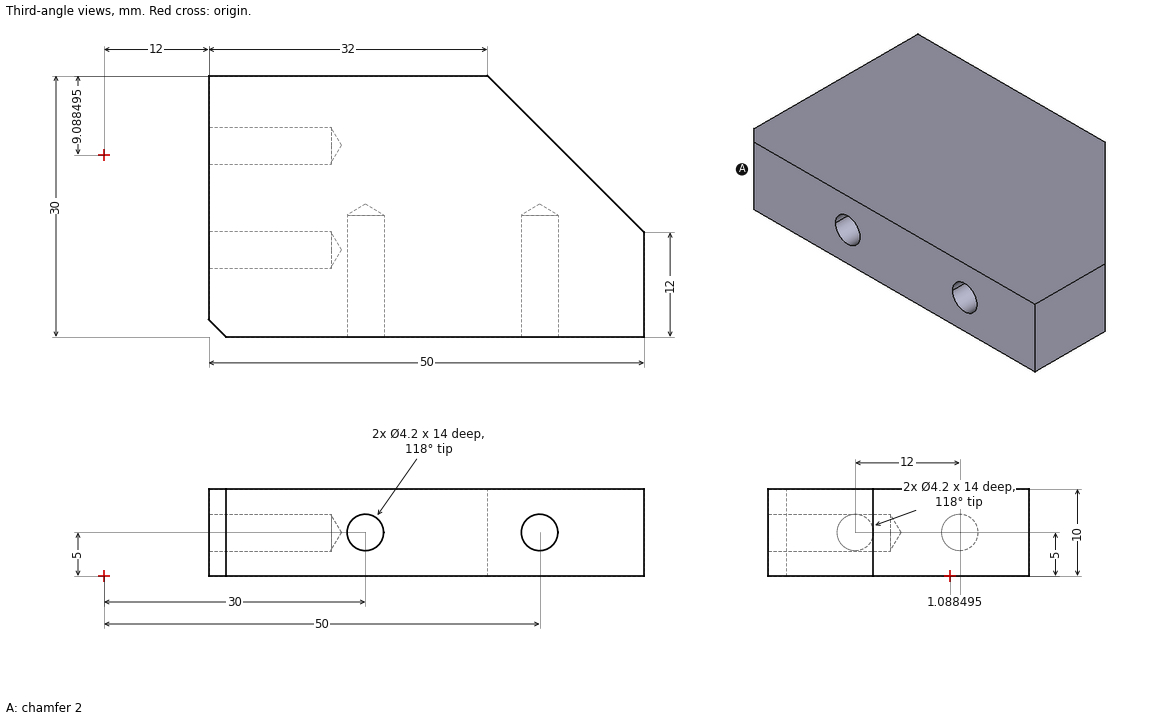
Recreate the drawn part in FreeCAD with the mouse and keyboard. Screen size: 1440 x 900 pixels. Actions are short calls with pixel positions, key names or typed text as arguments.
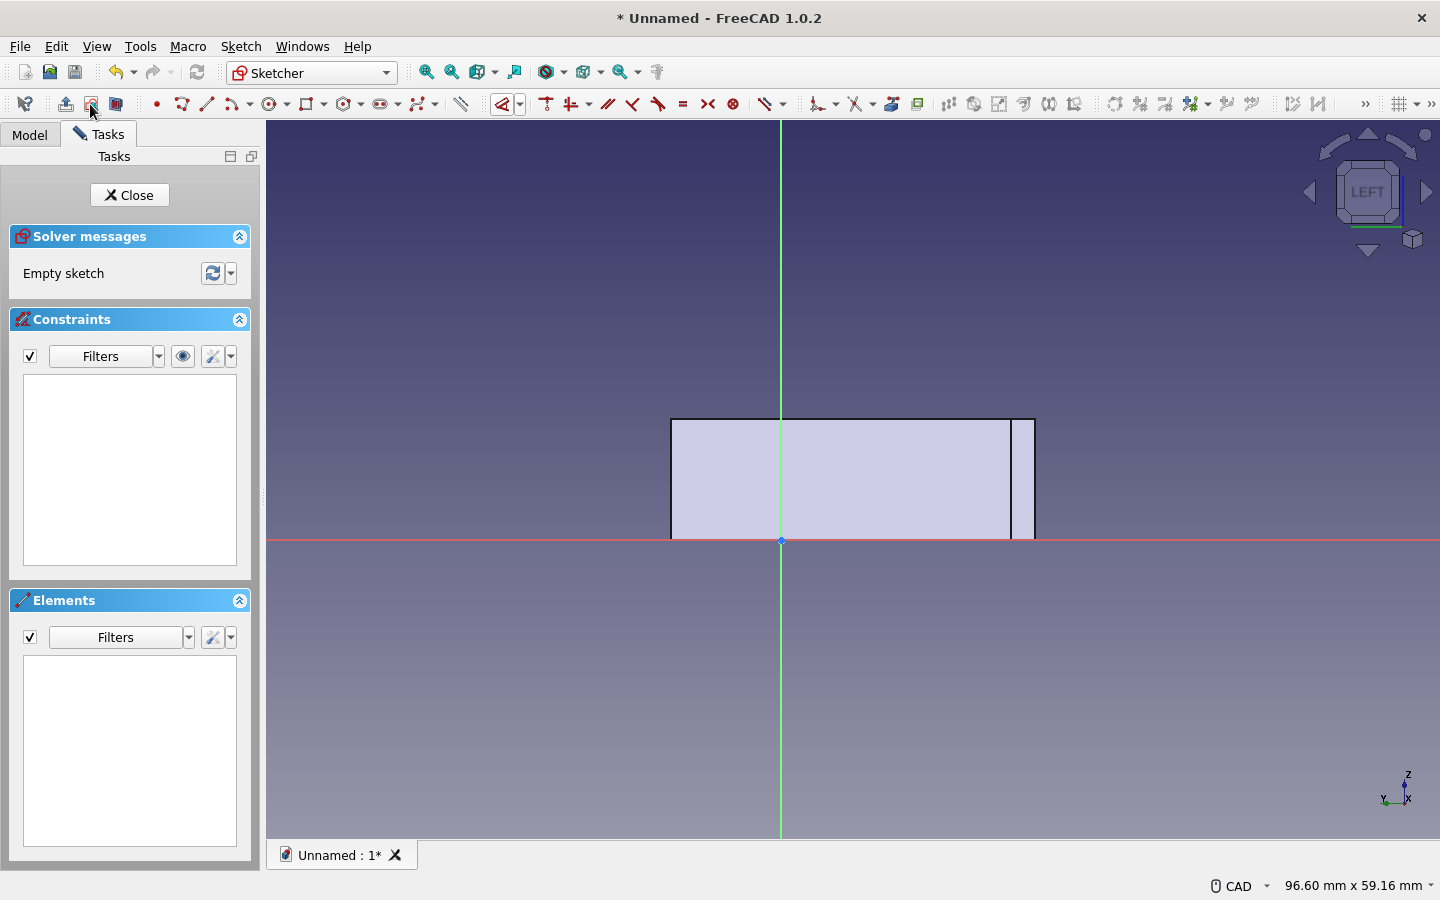
scroll(865, 505, up, 6)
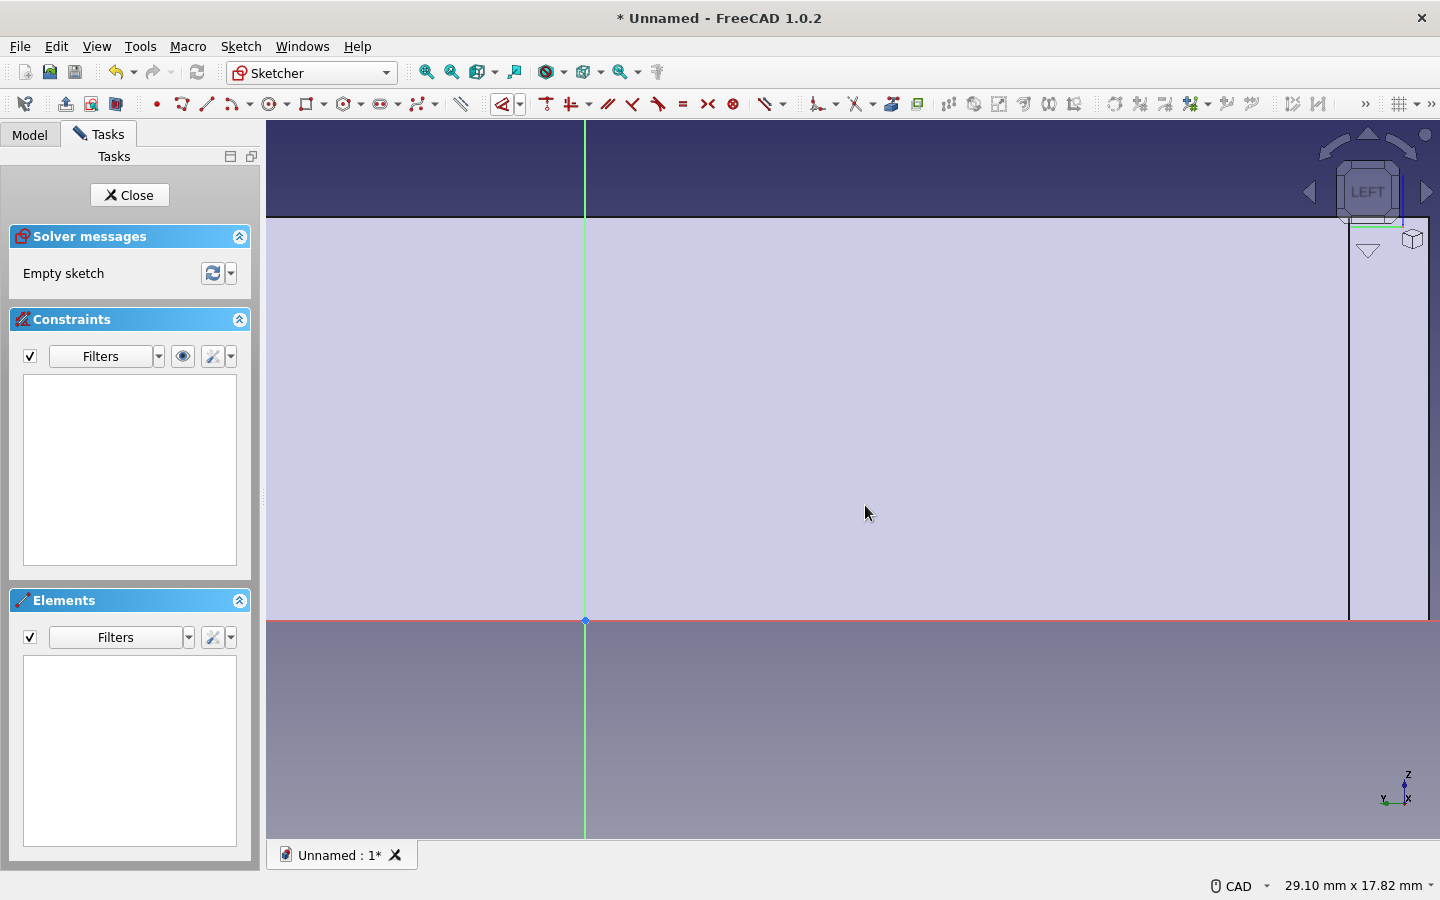
click(268, 104)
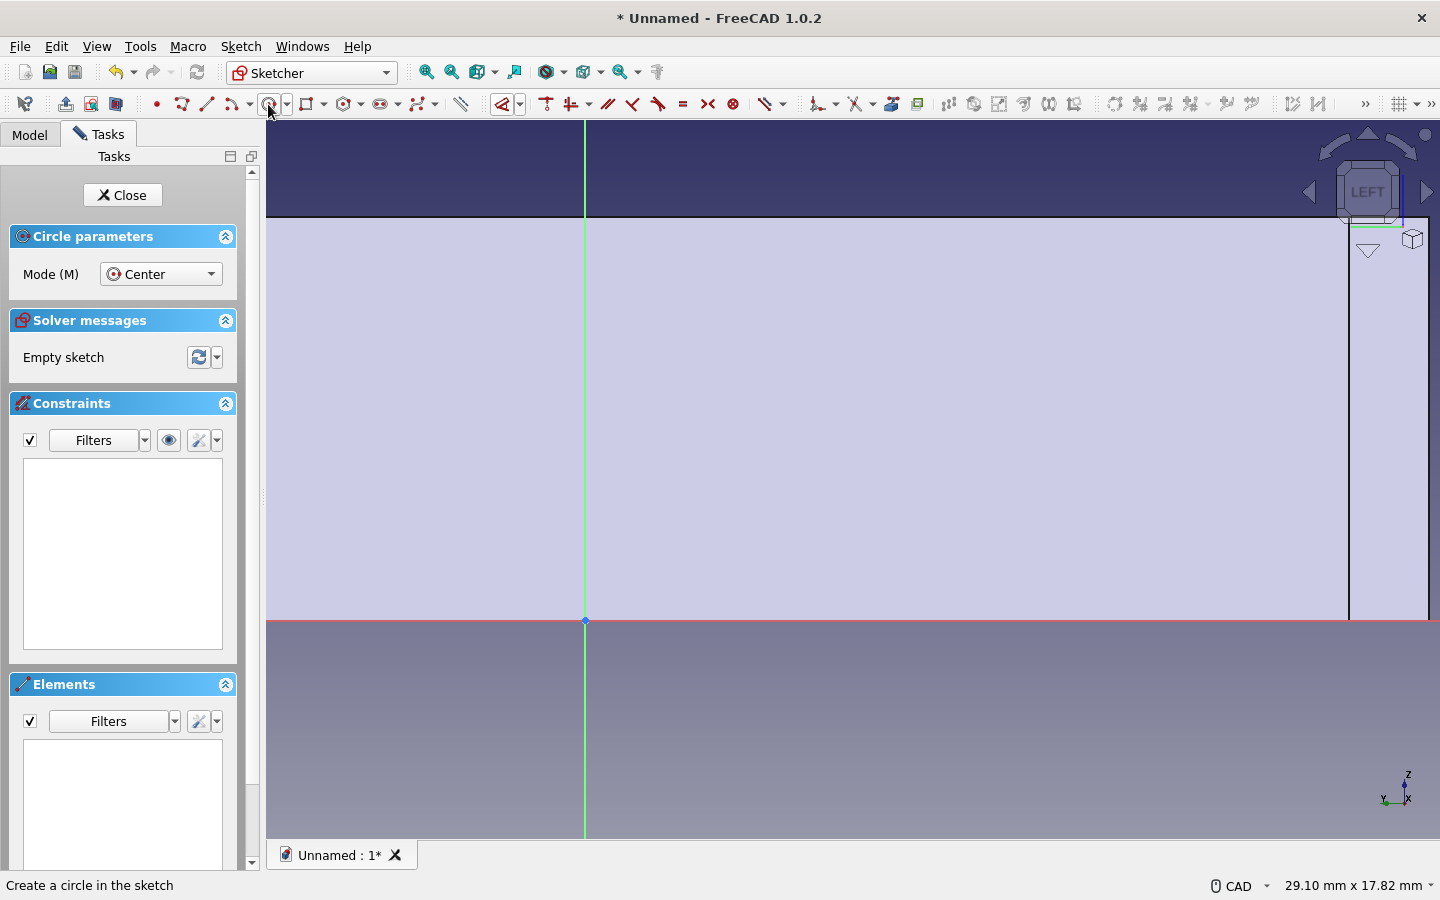
click(1026, 419)
move(1086, 359)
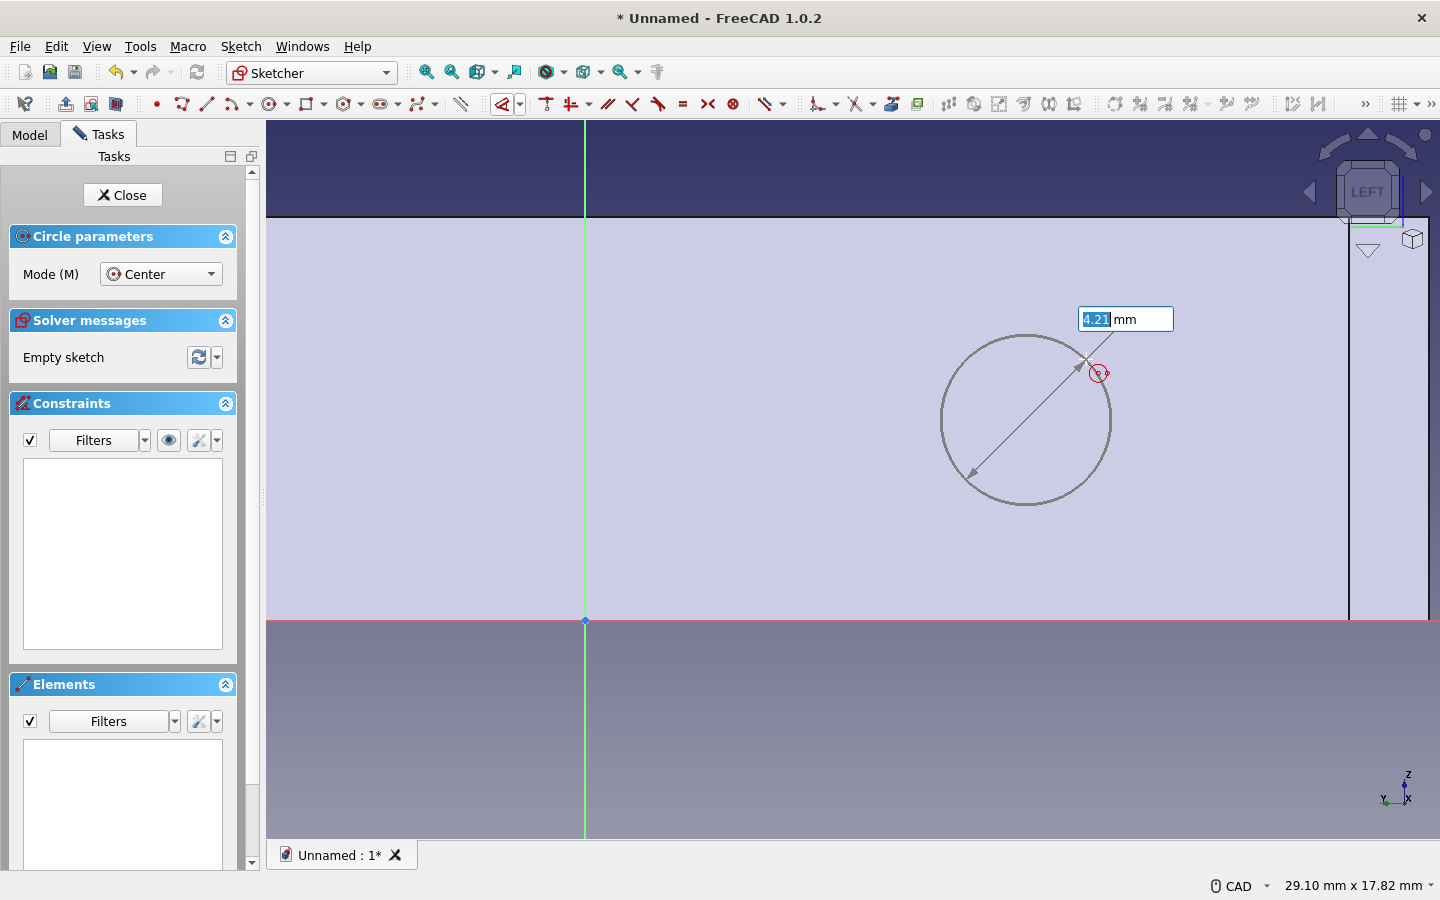
text(4.2)
key(Return)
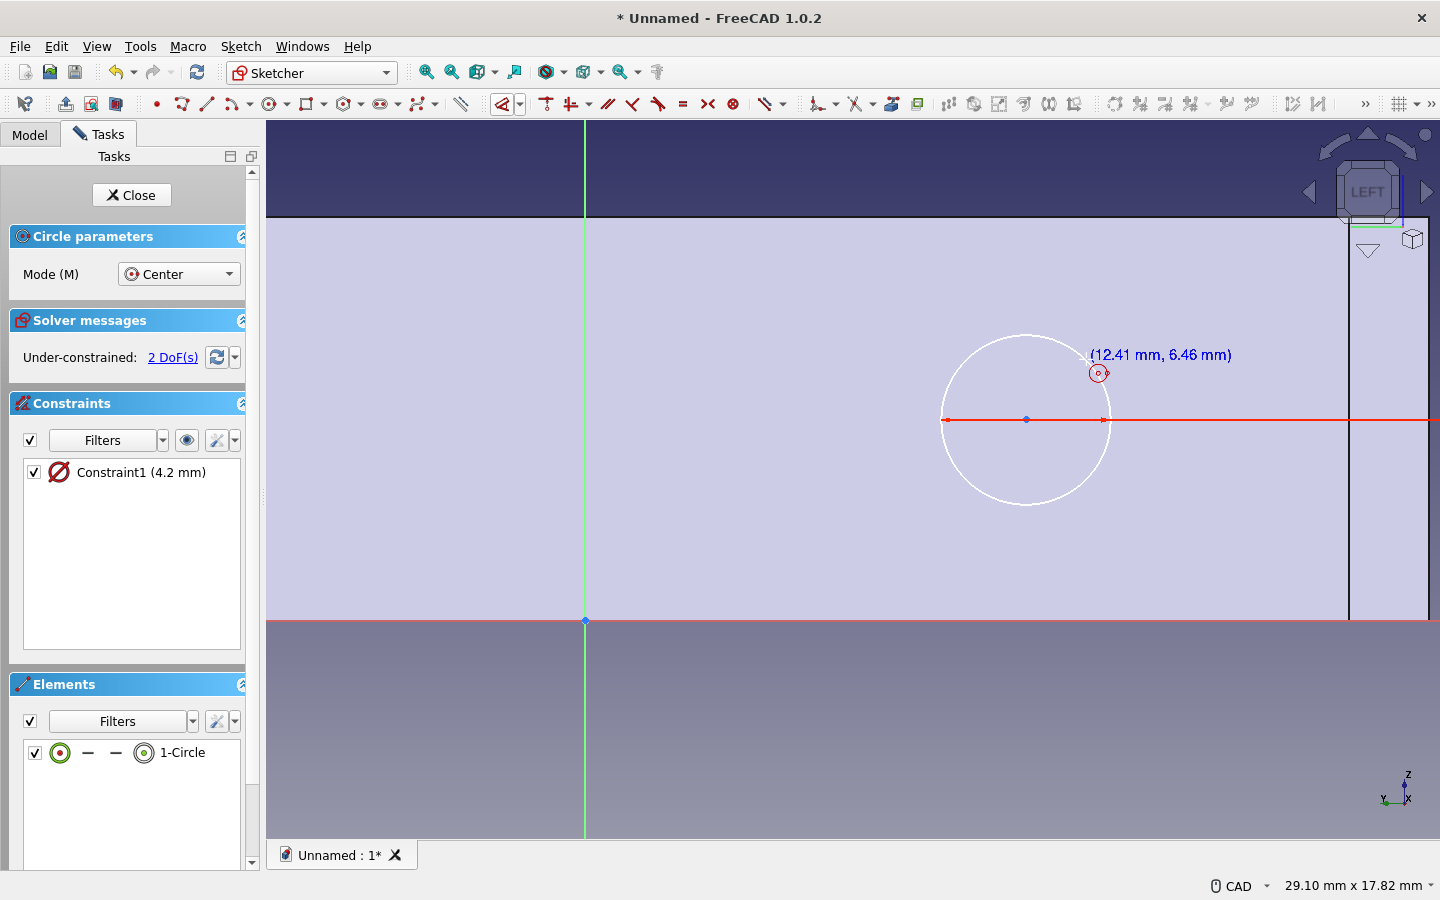
click(542, 419)
move(601, 359)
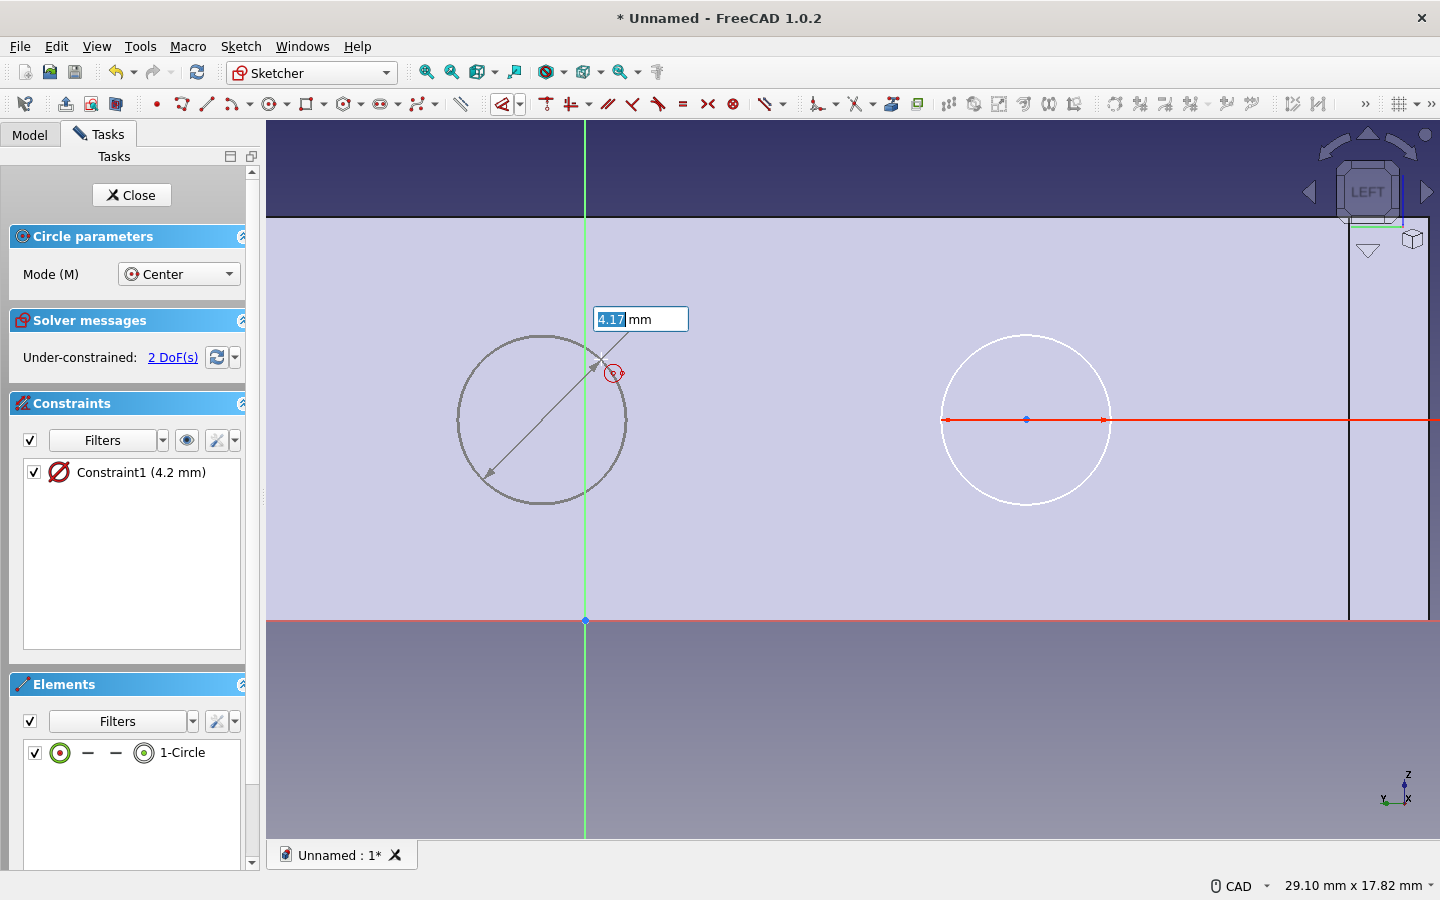
text(4.2)
key(Return)
key(Escape)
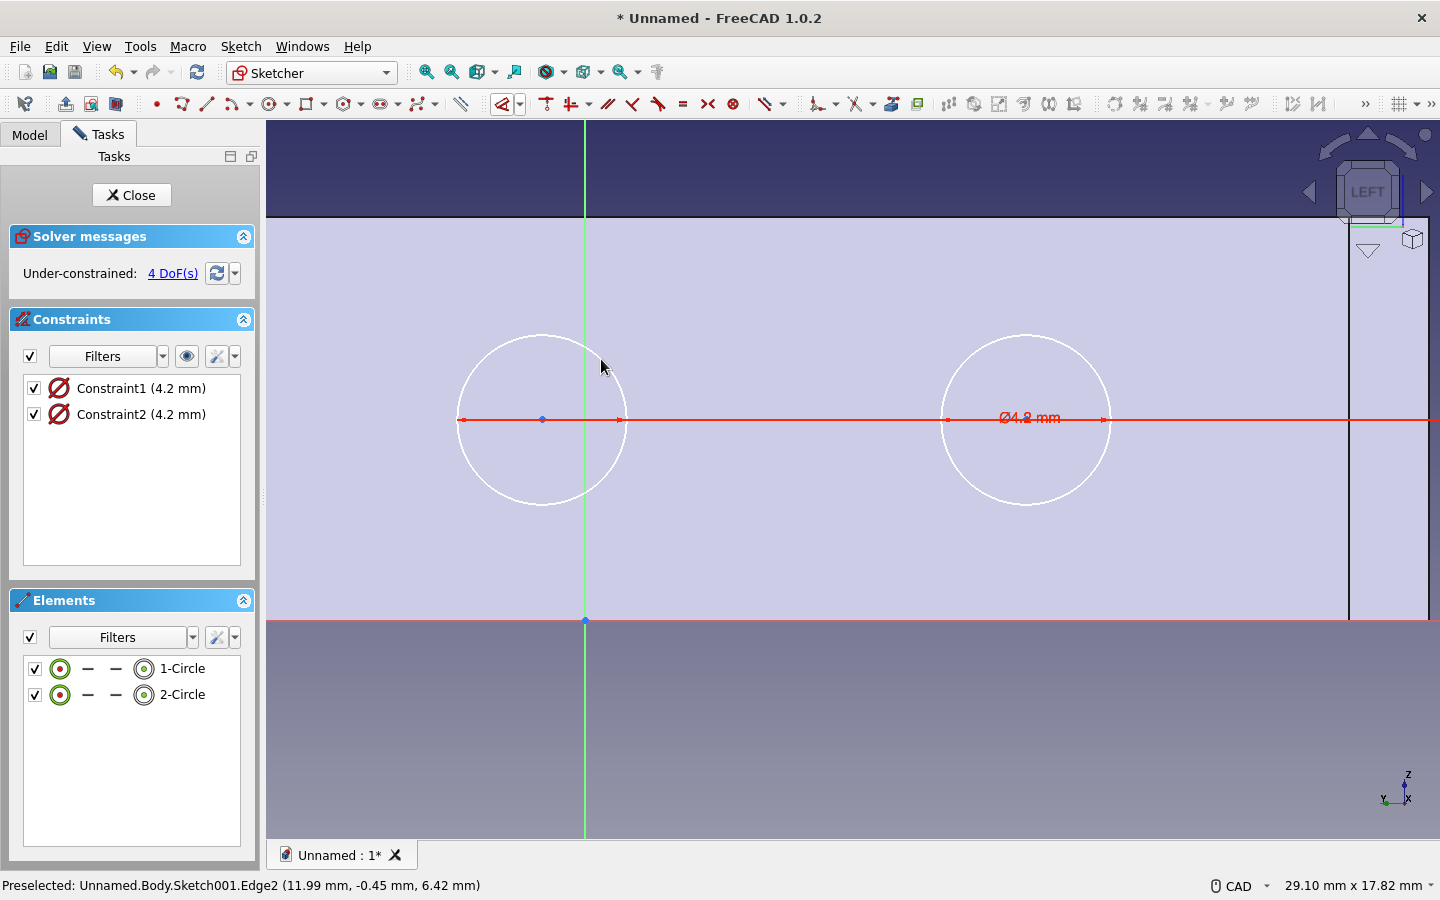
click(1026, 420)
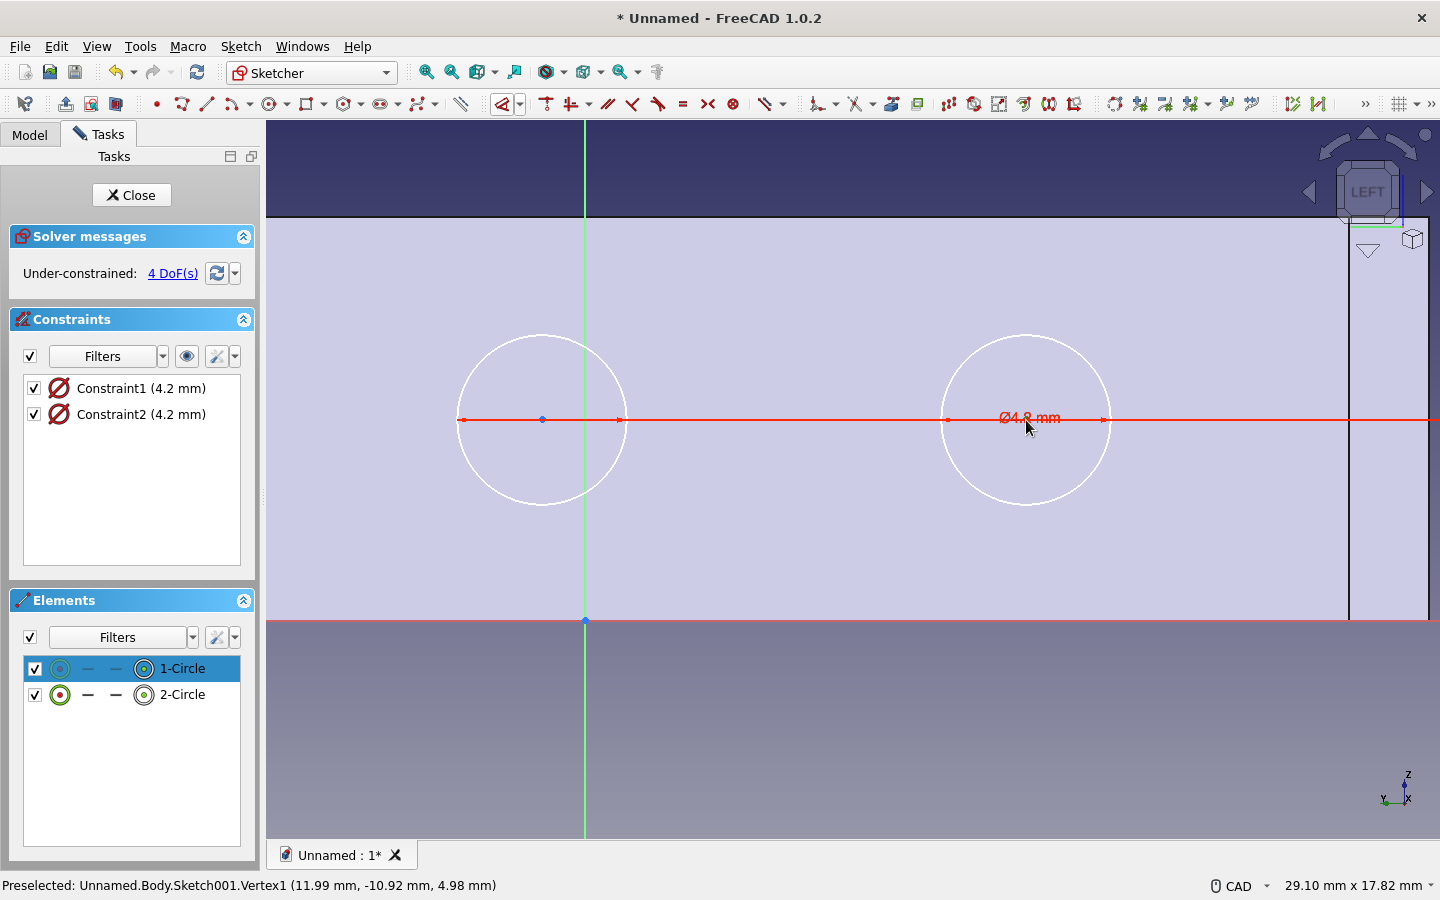
click(542, 420)